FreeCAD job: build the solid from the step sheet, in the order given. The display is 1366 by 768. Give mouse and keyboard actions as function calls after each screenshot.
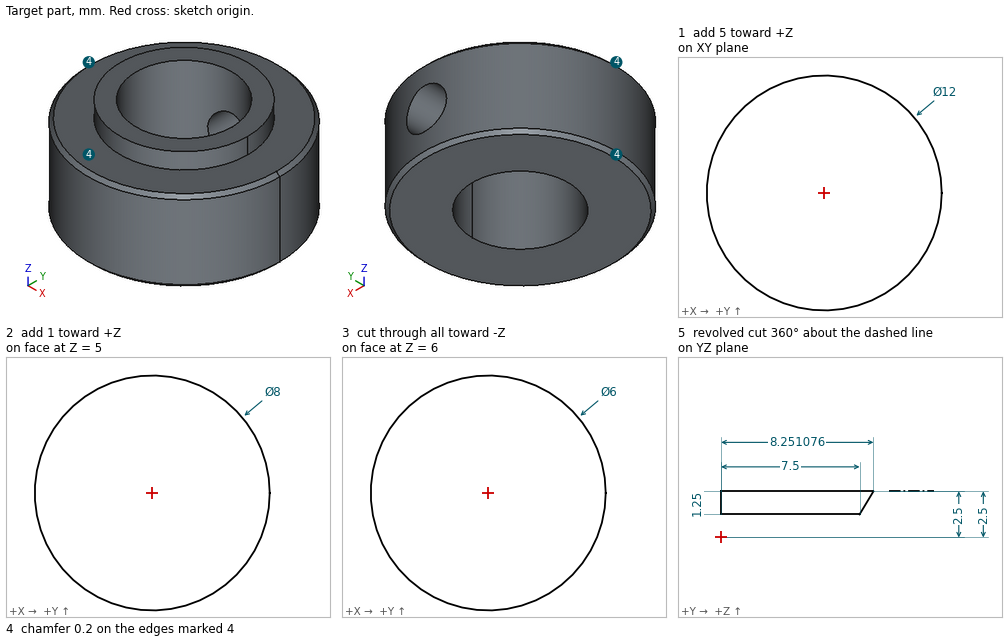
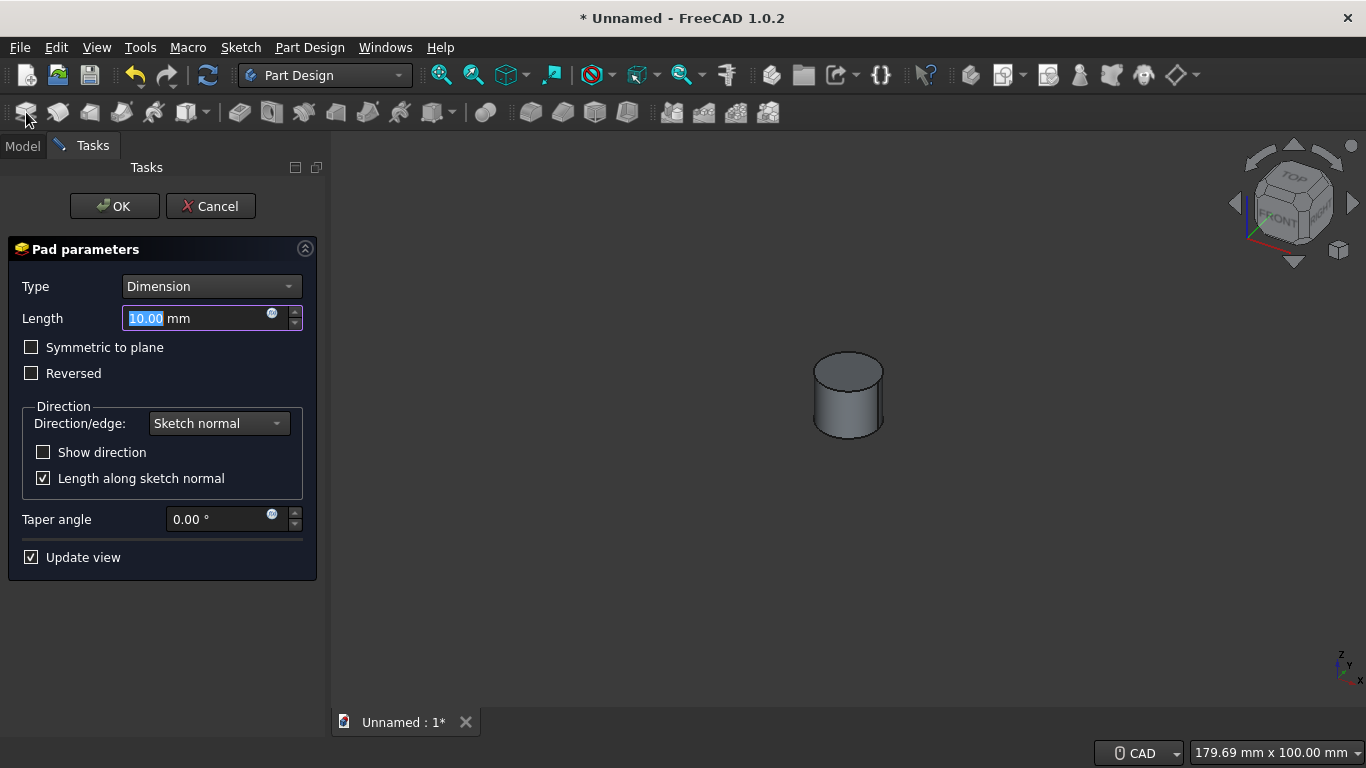
text(5)
key(Tab)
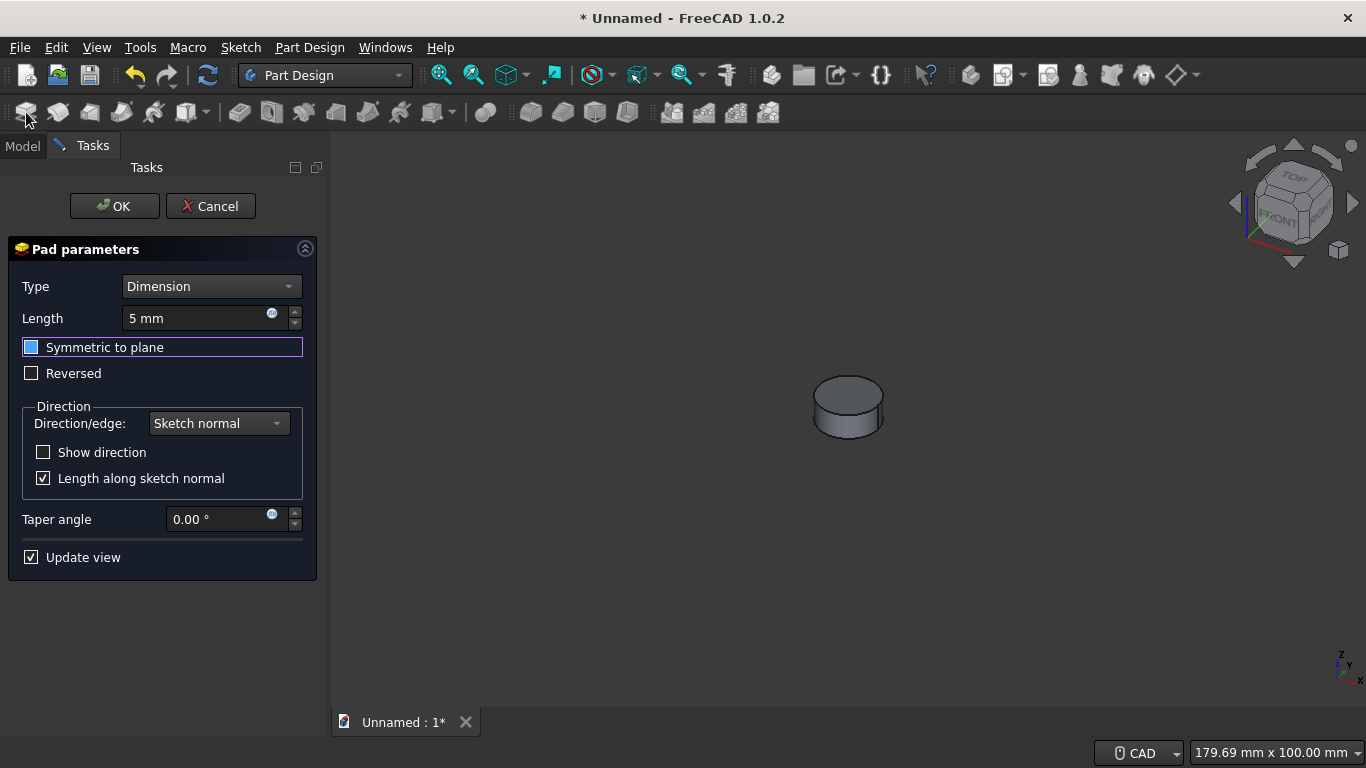
click(115, 206)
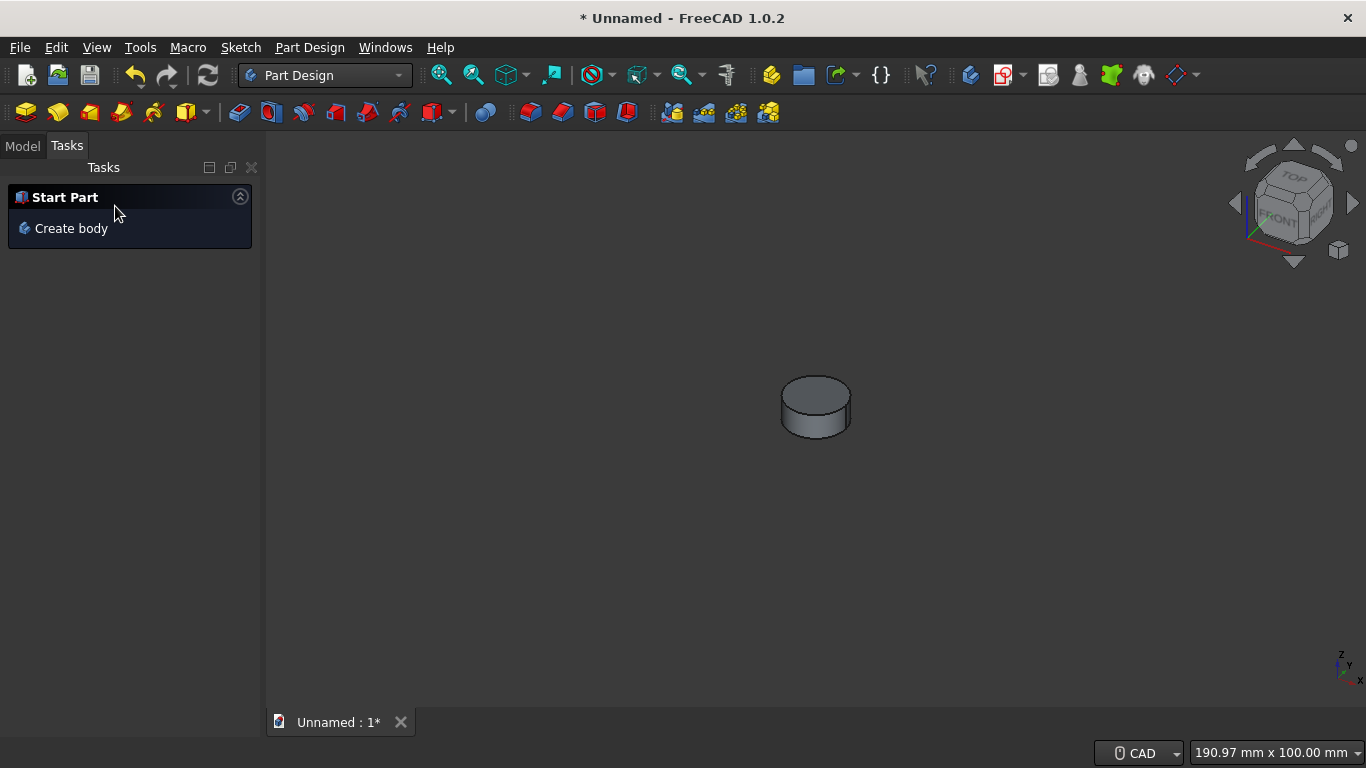
click(442, 76)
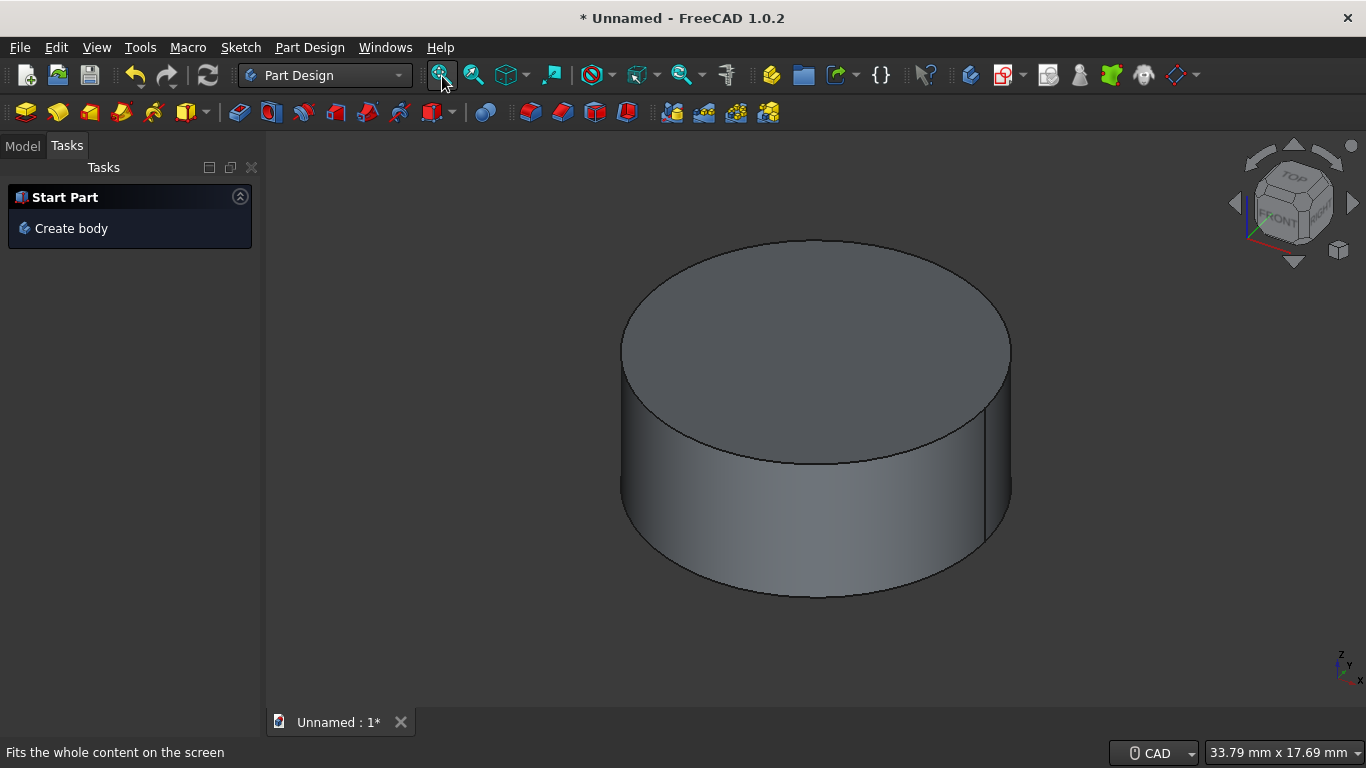
click(816, 351)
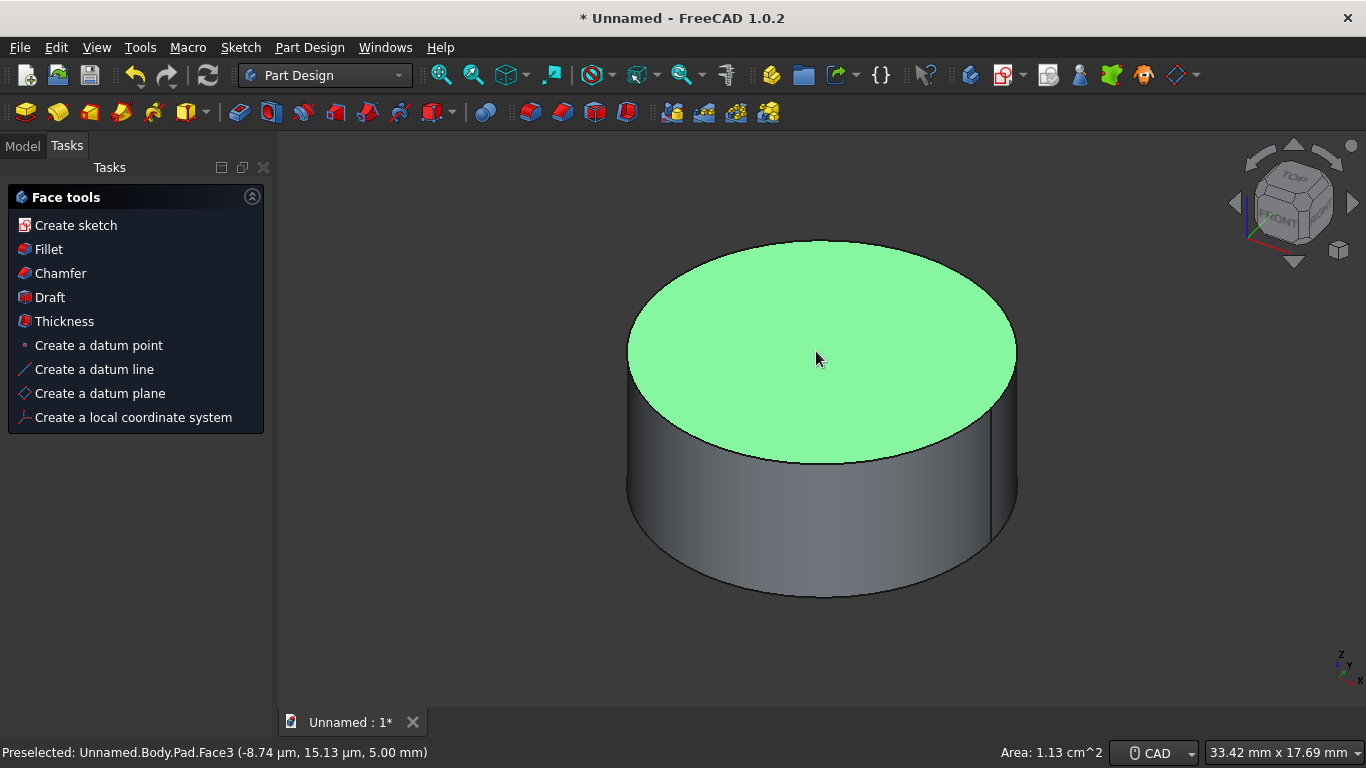
click(1004, 76)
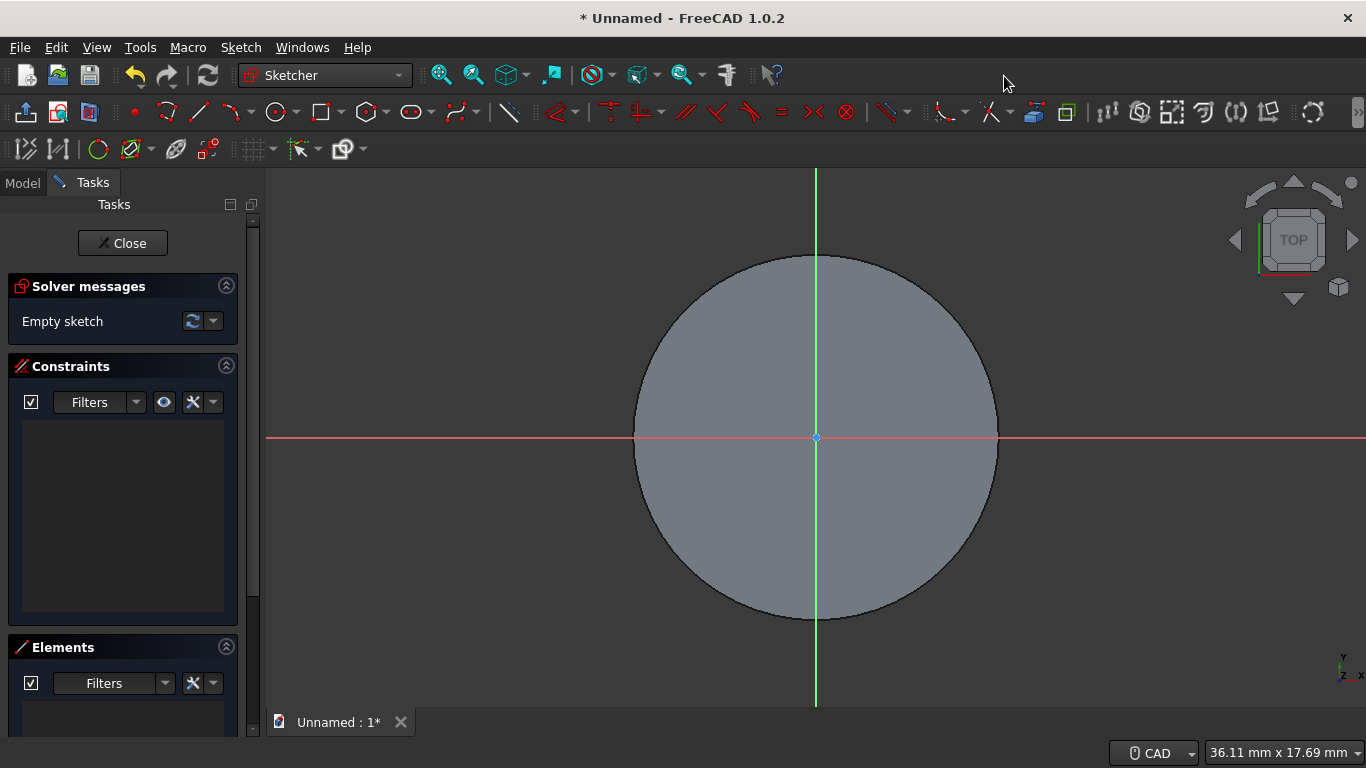
scroll(955, 438, up, 2)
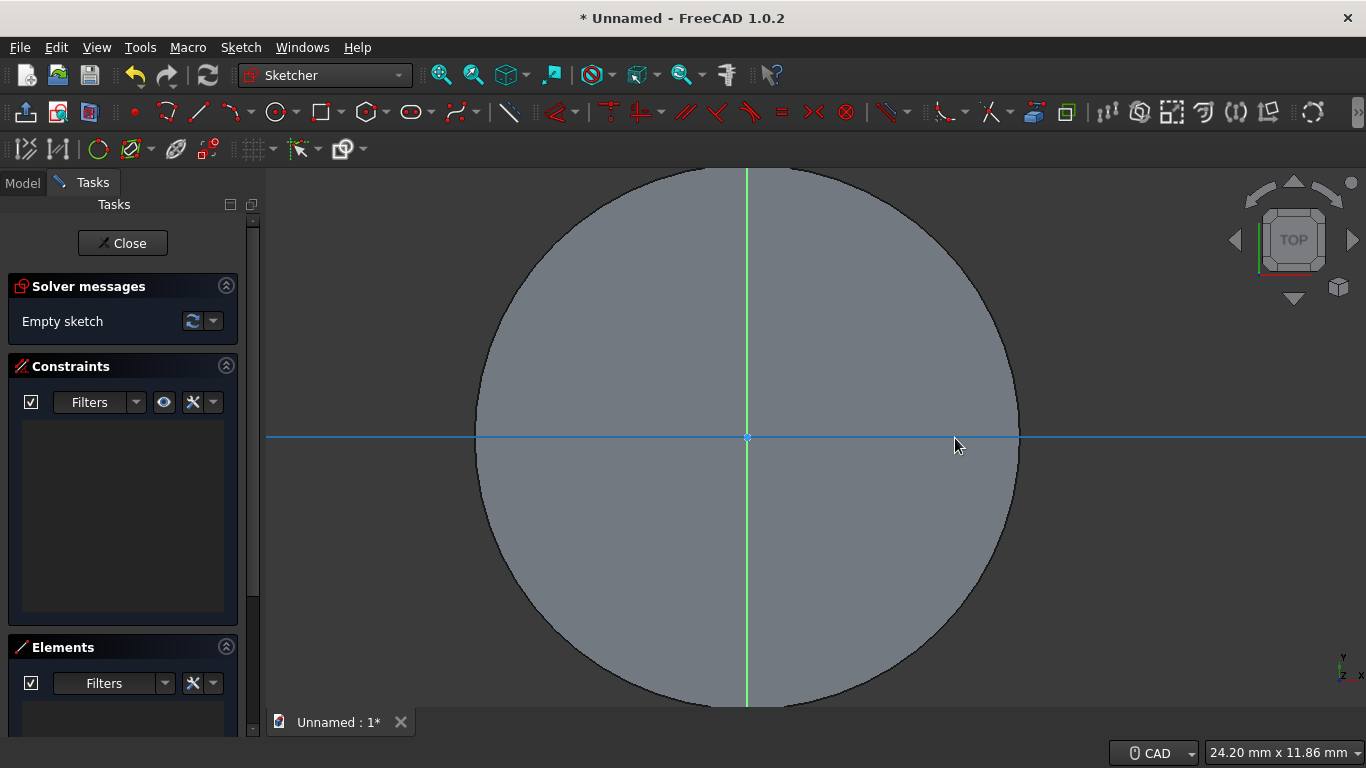
click(276, 112)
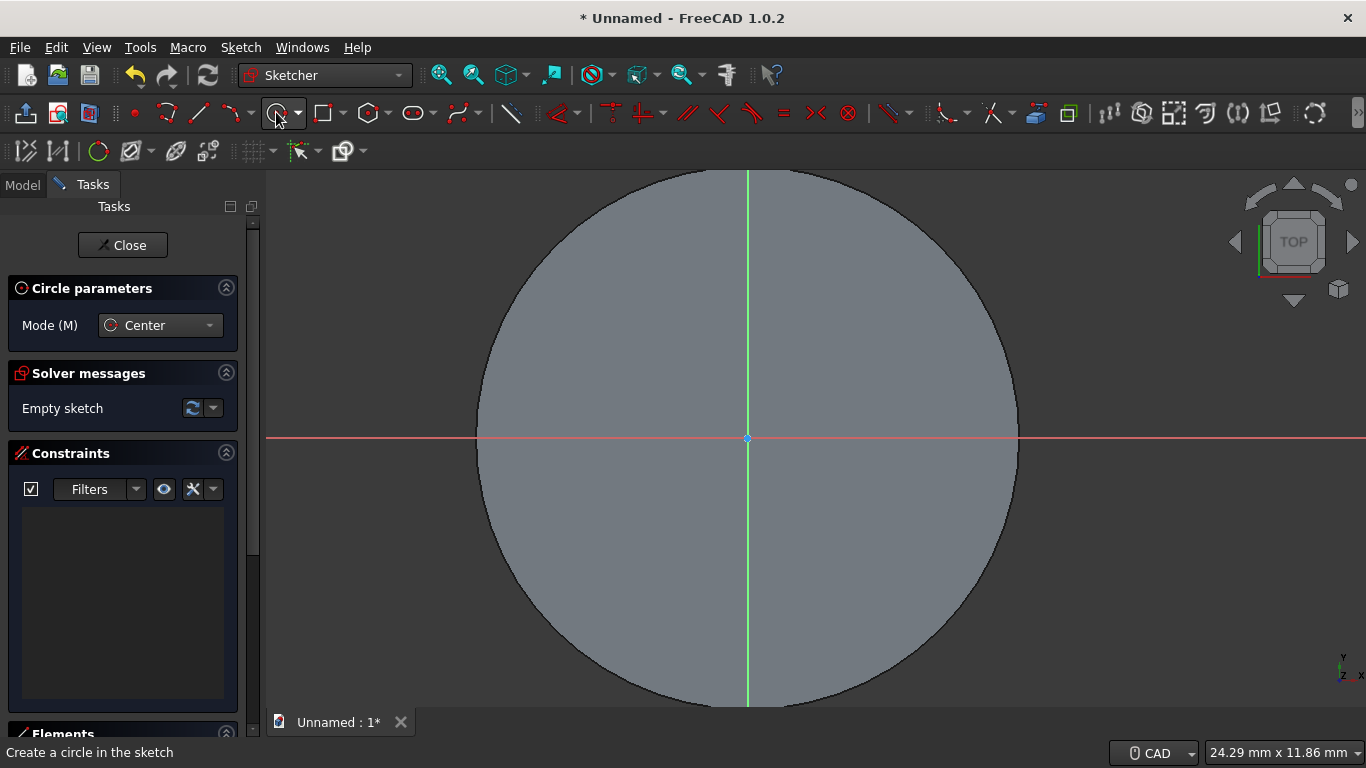
click(748, 438)
move(876, 310)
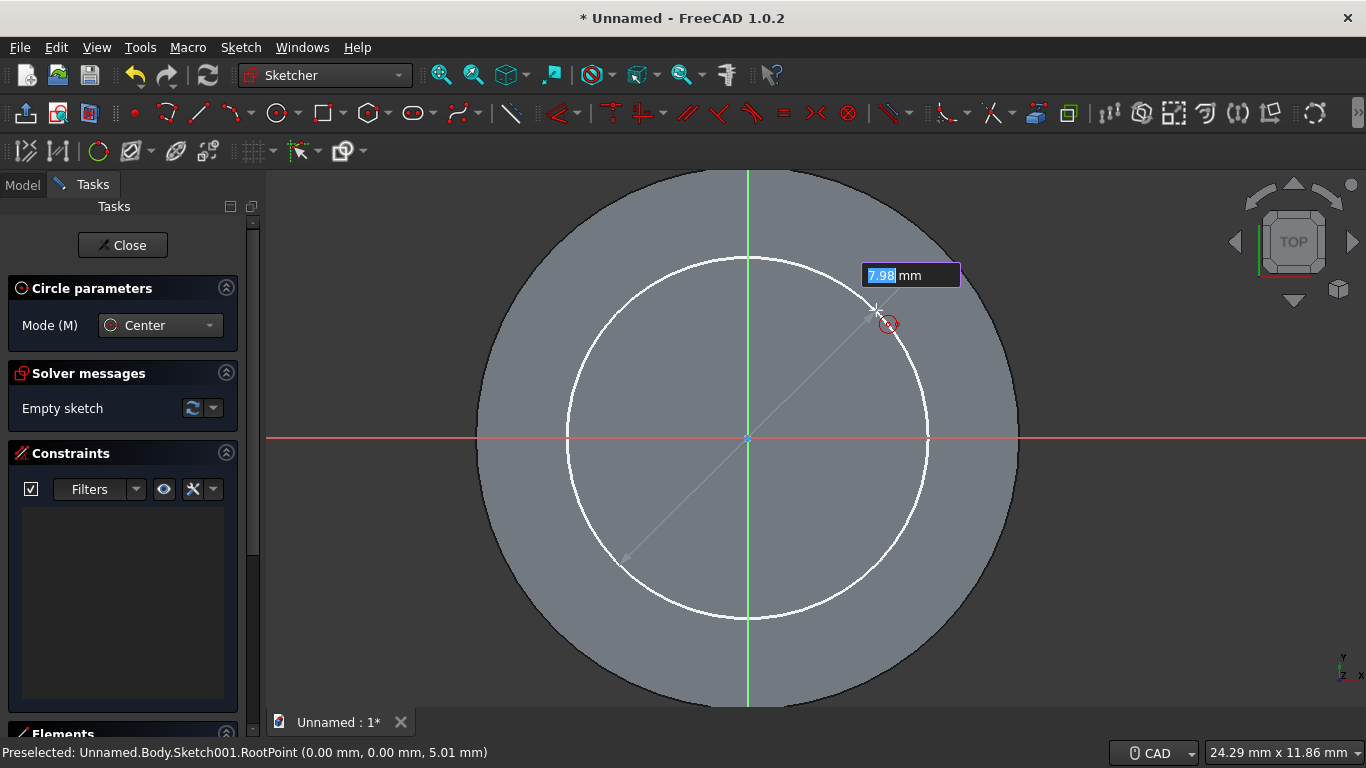
text(8)
key(Return)
key(Escape)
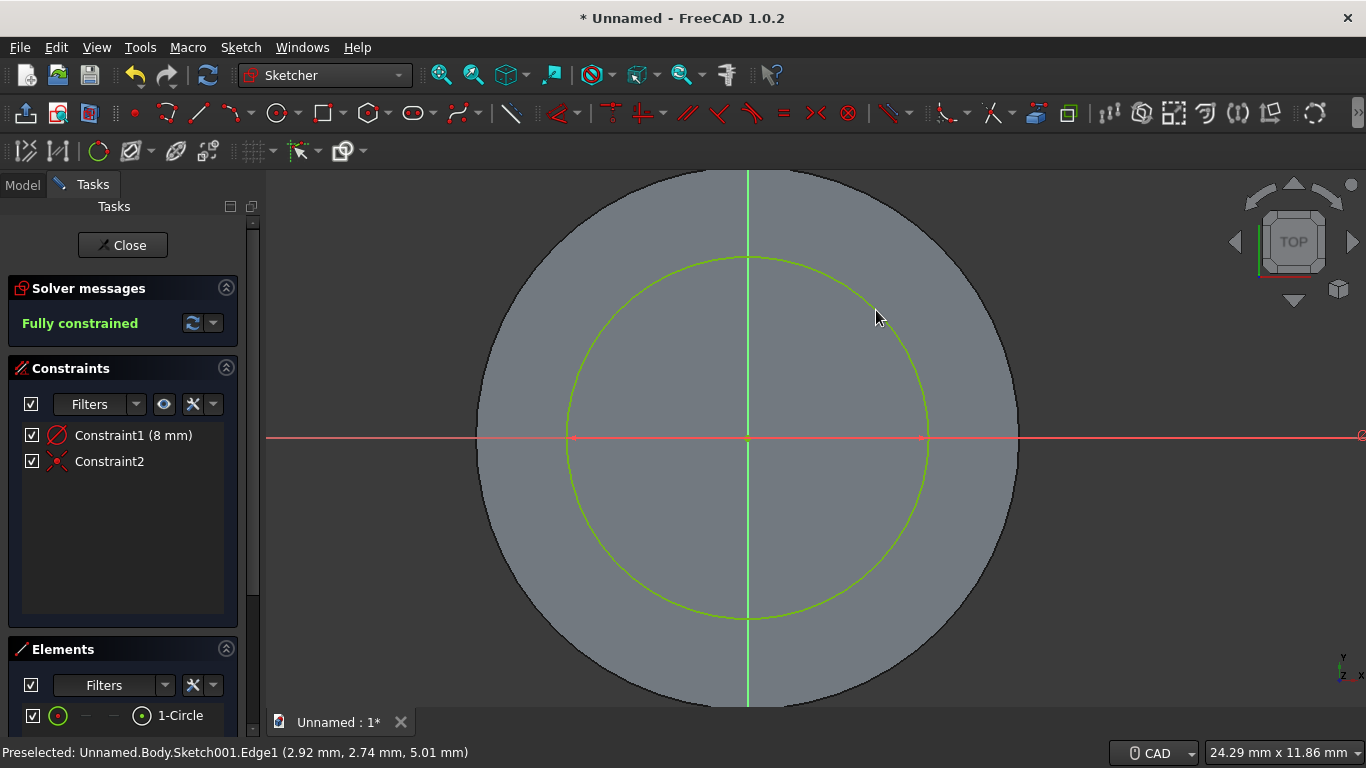
click(123, 245)